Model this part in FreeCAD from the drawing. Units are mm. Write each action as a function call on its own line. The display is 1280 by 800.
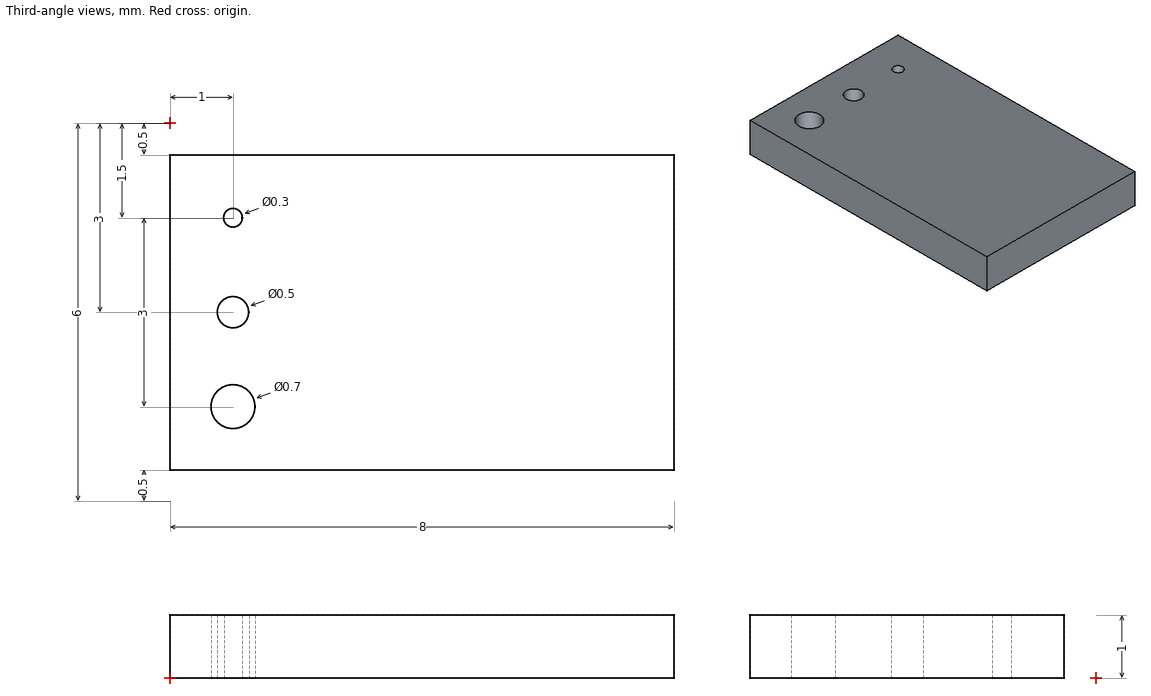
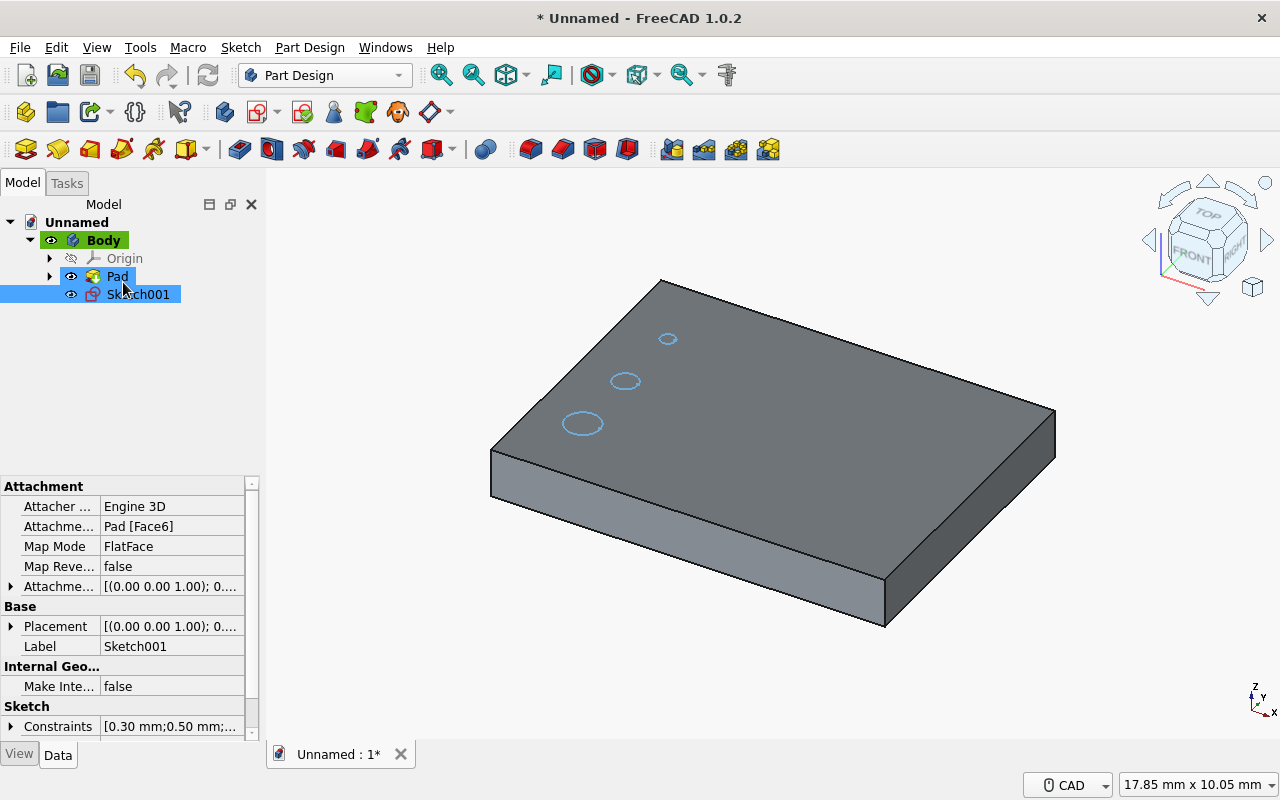
click(240, 150)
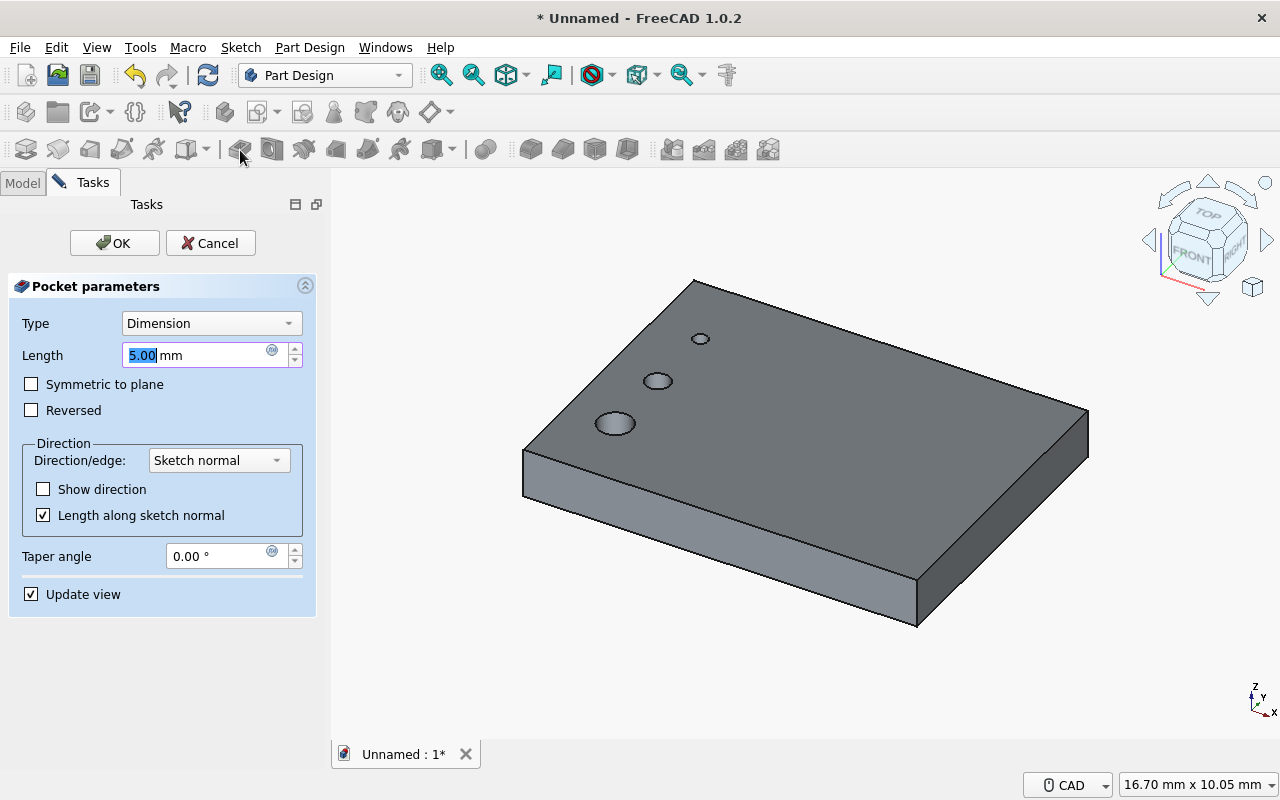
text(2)
key(Tab)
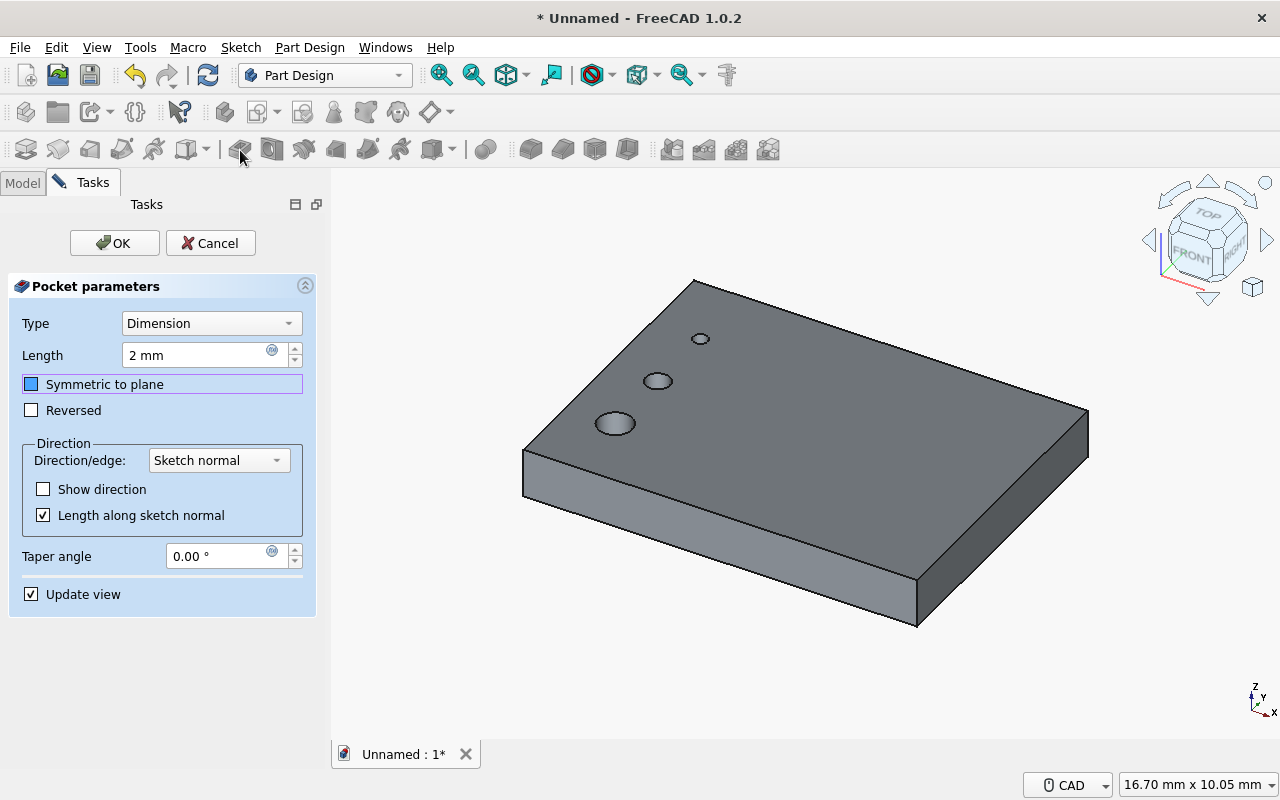
click(115, 243)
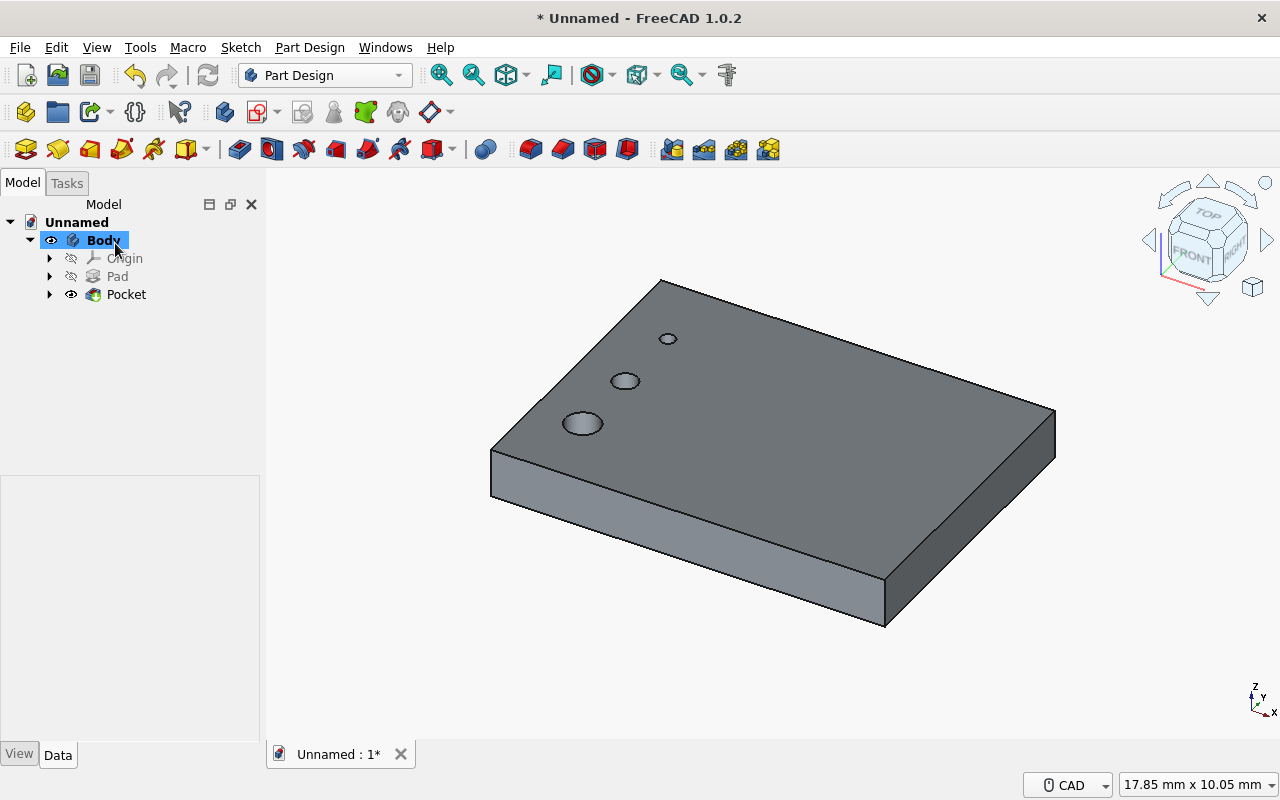
click(829, 448)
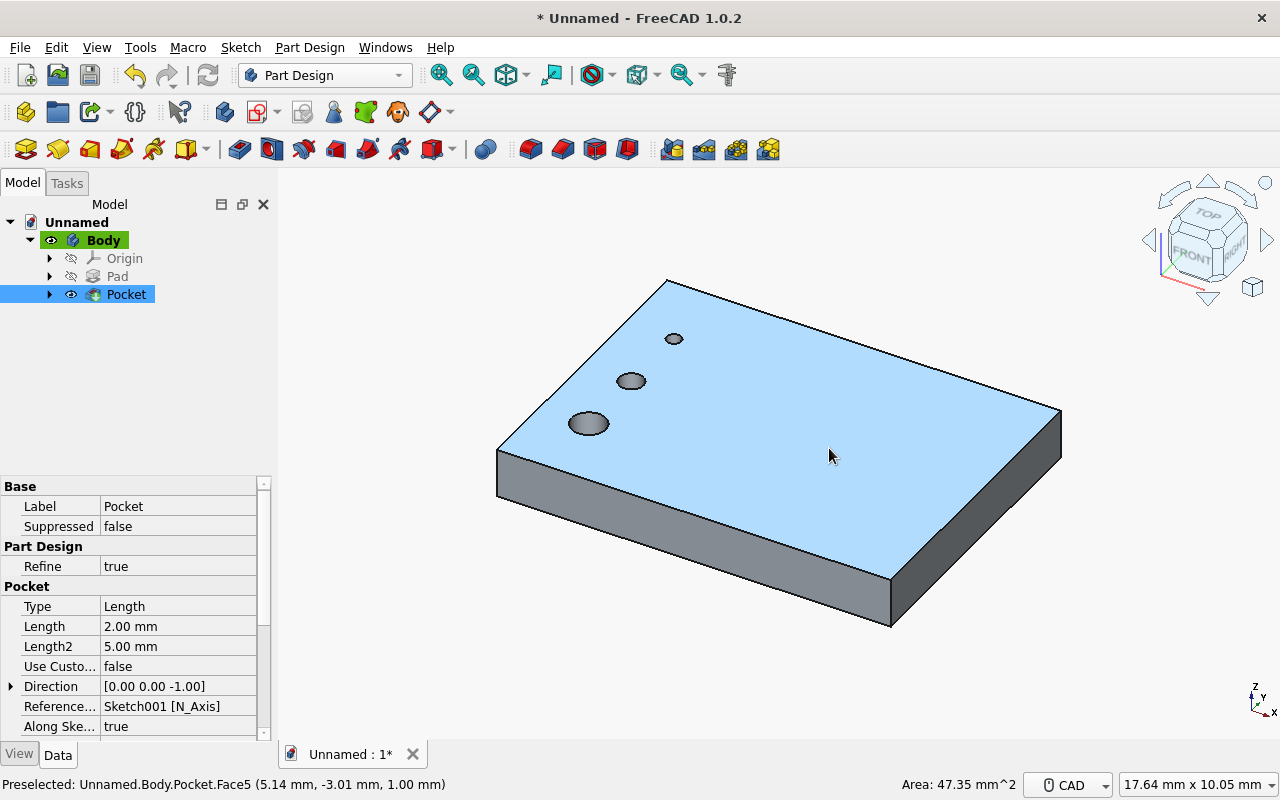
click(258, 112)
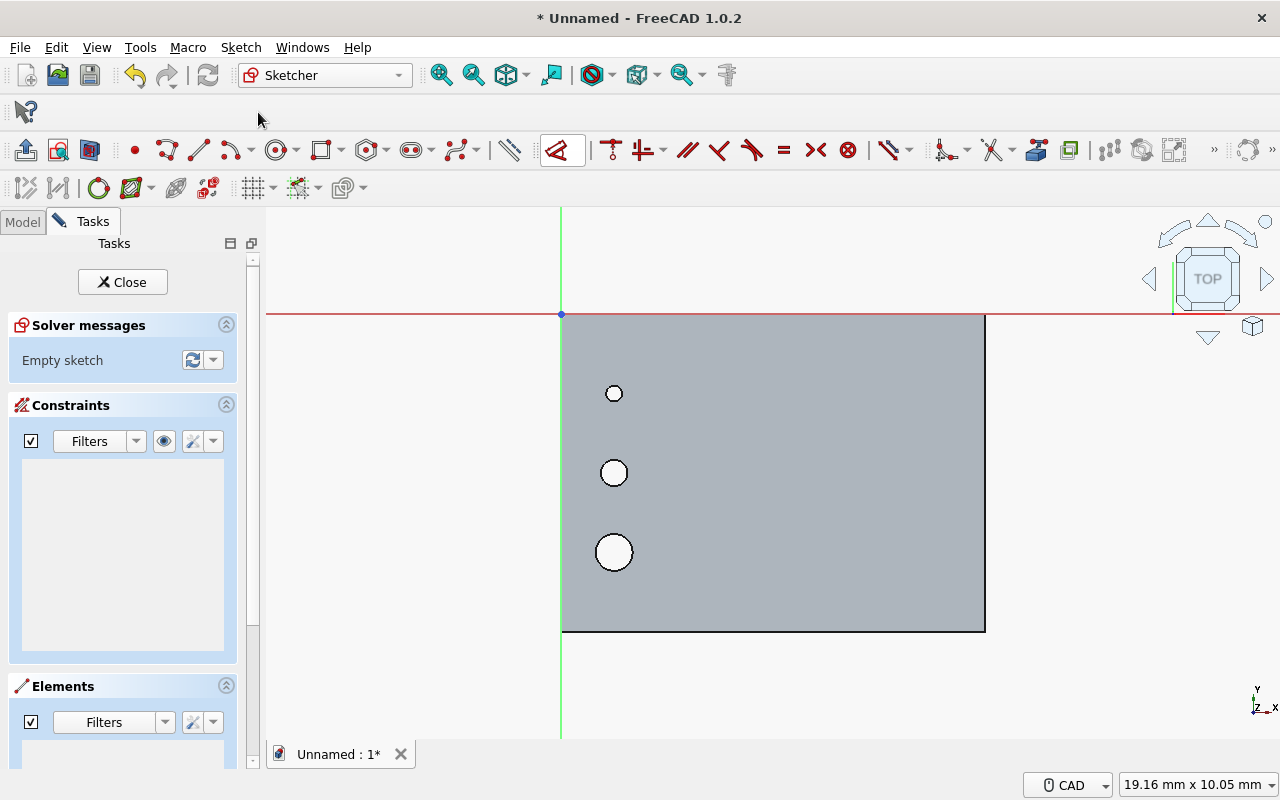
key(g)
key(r)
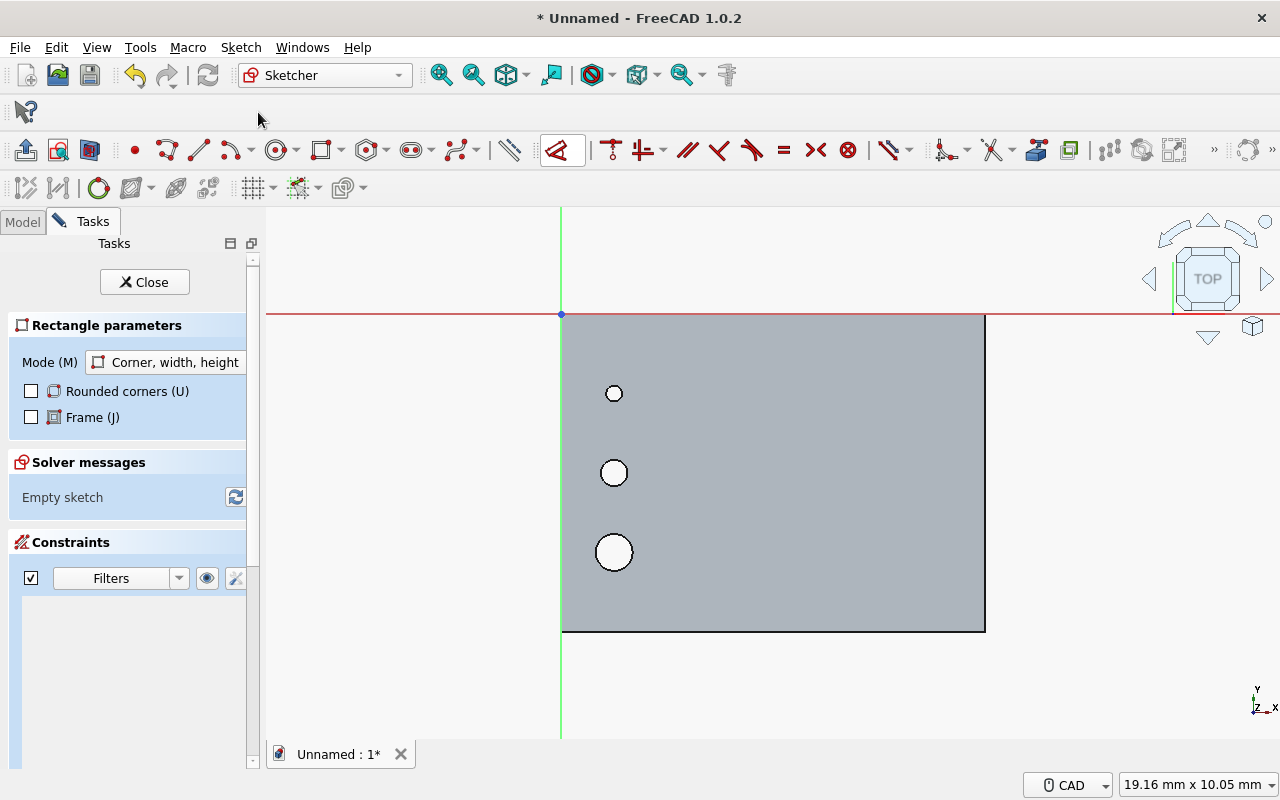
click(561, 314)
click(985, 341)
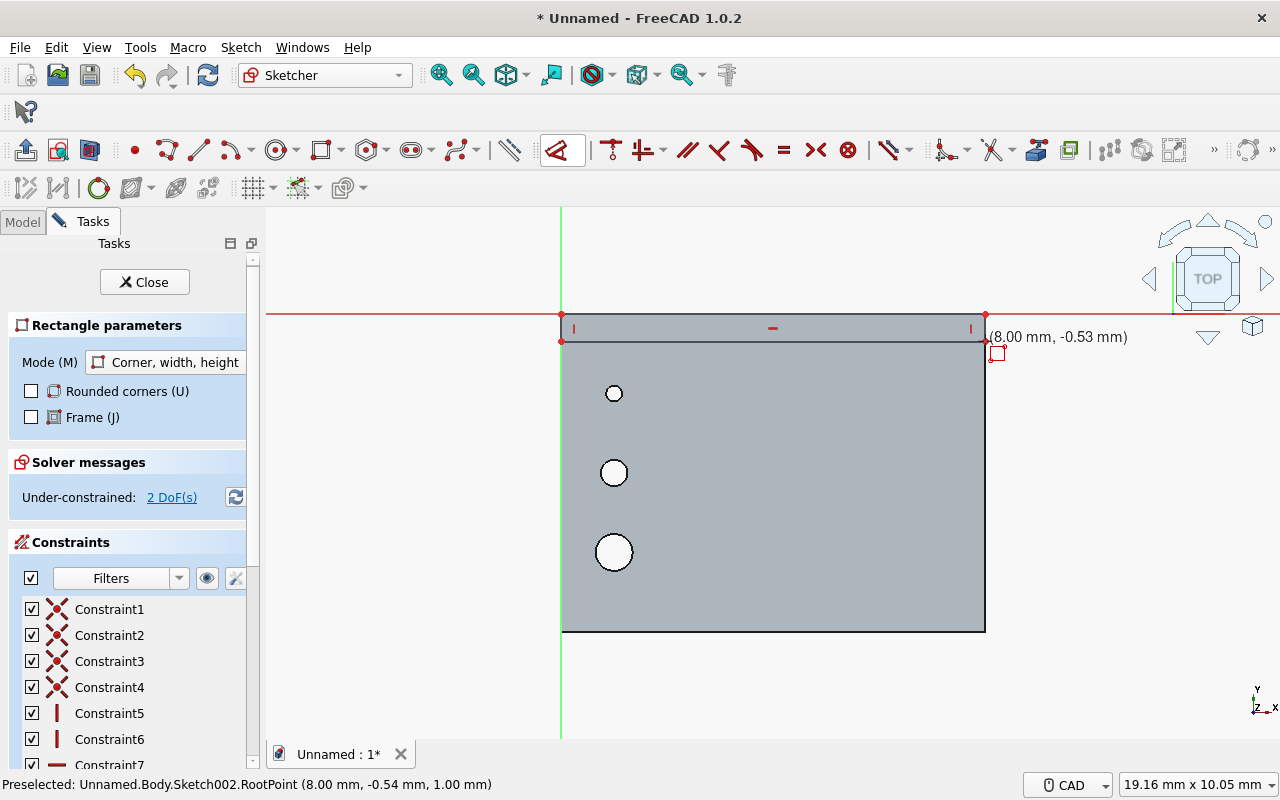
click(561, 605)
click(985, 632)
key(Escape)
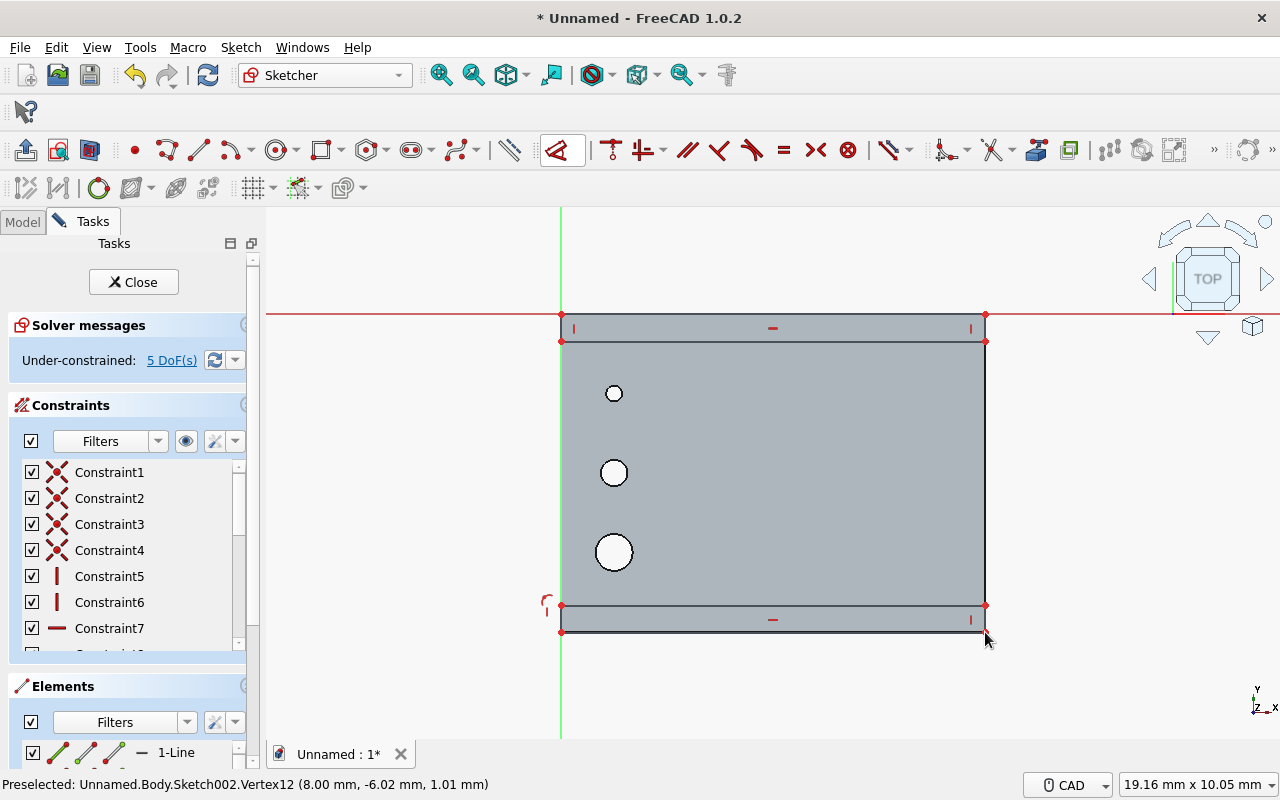
click(688, 342)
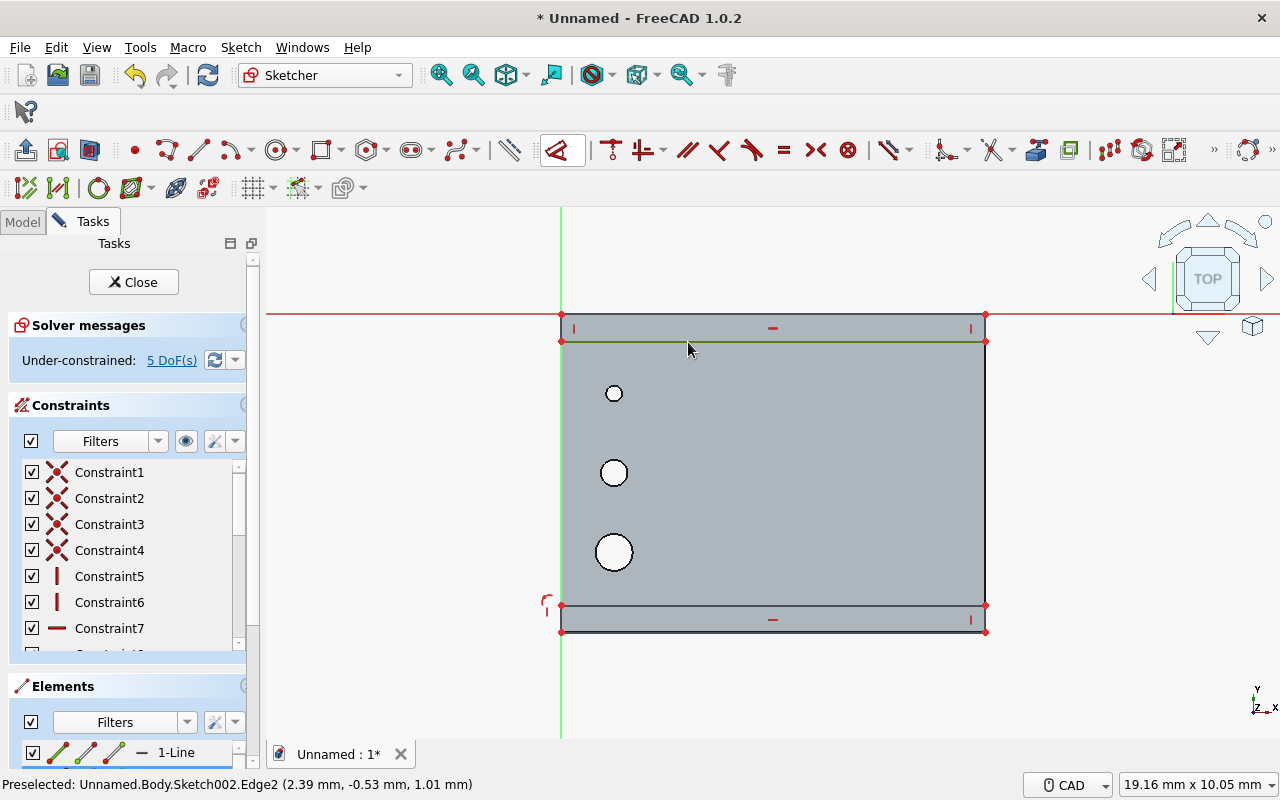
click(580, 150)